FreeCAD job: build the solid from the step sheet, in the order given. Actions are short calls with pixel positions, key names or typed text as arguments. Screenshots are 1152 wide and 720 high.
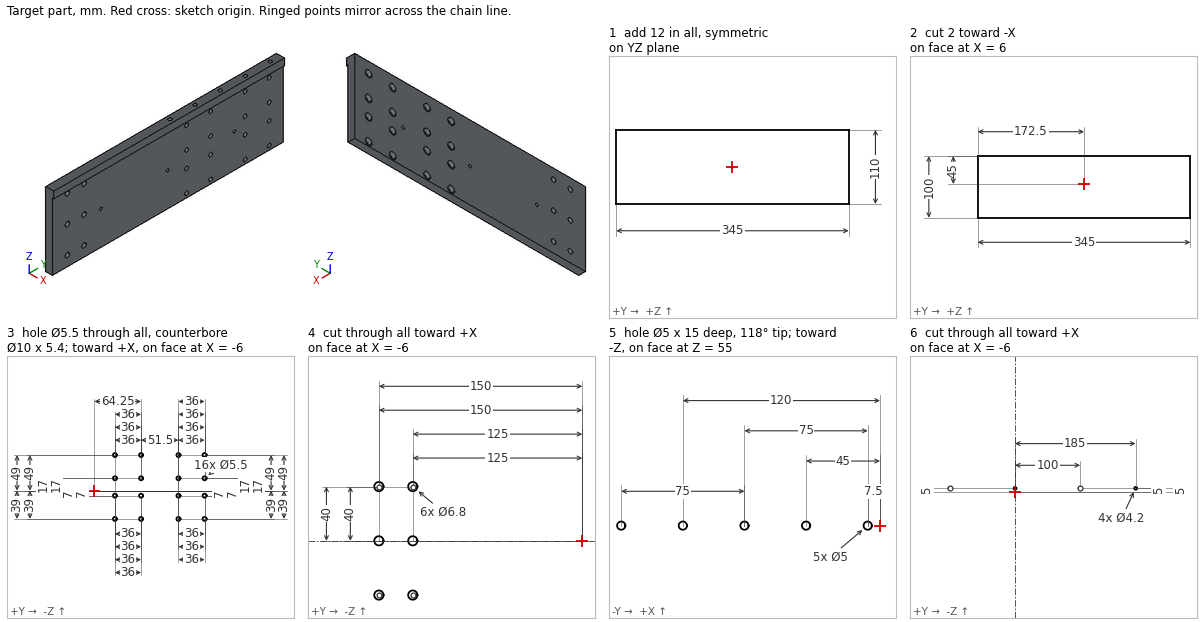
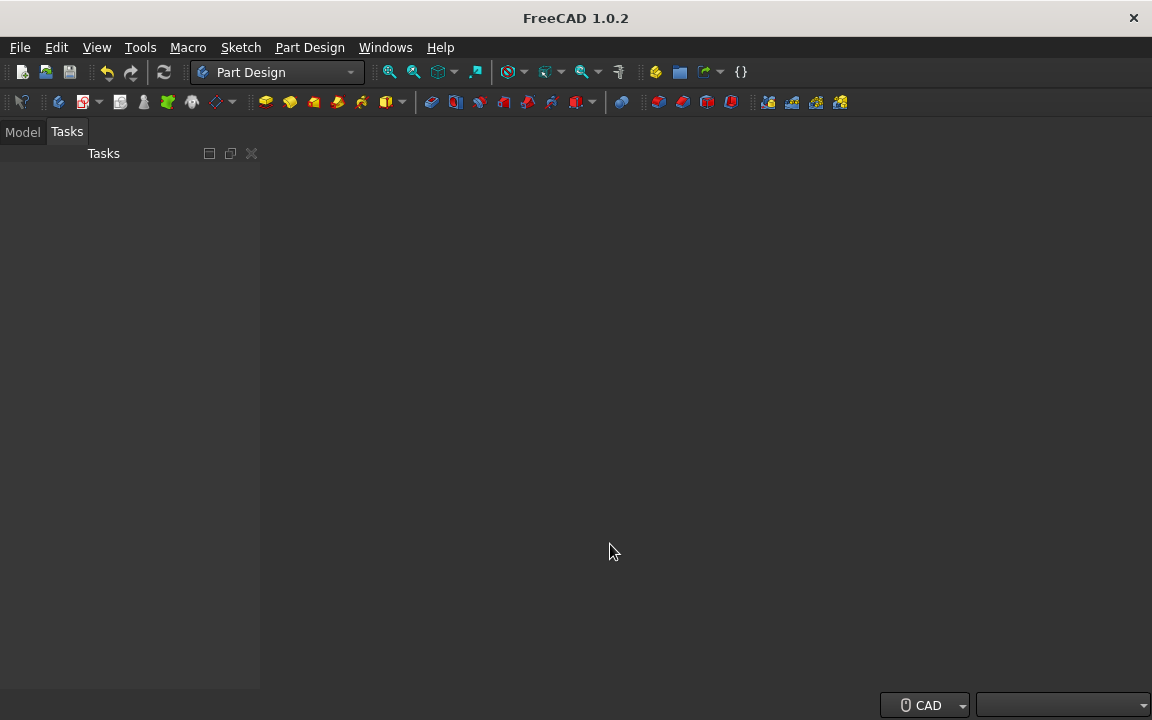
click(22, 72)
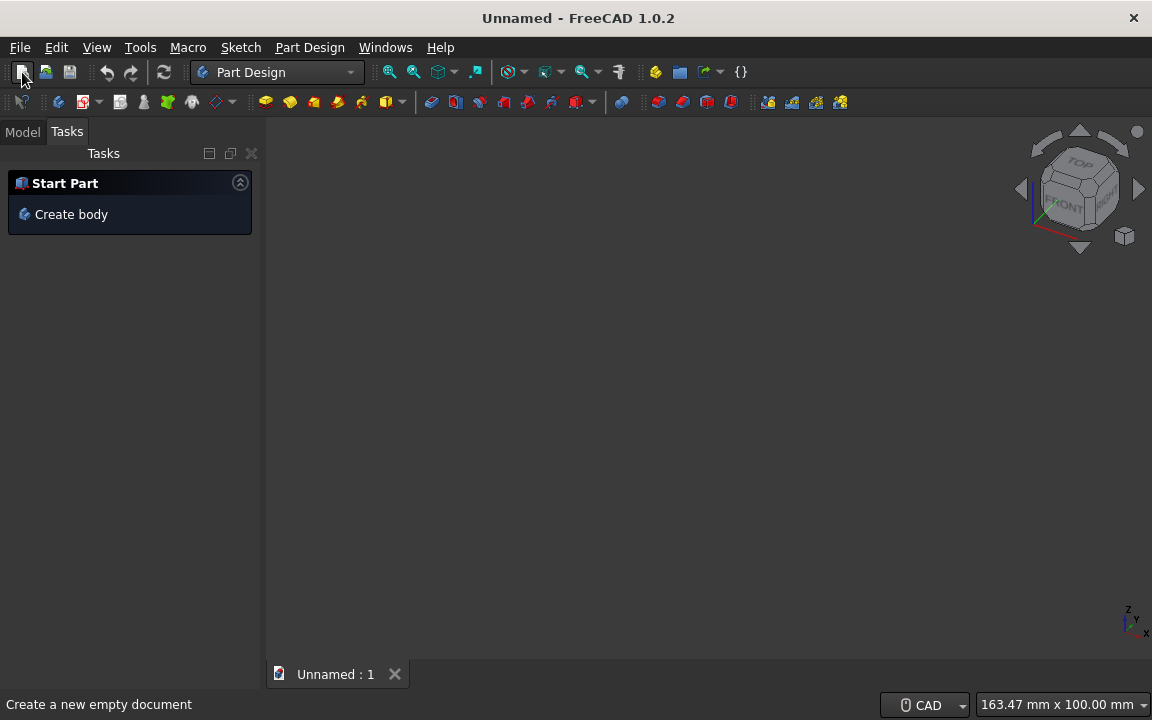
click(84, 102)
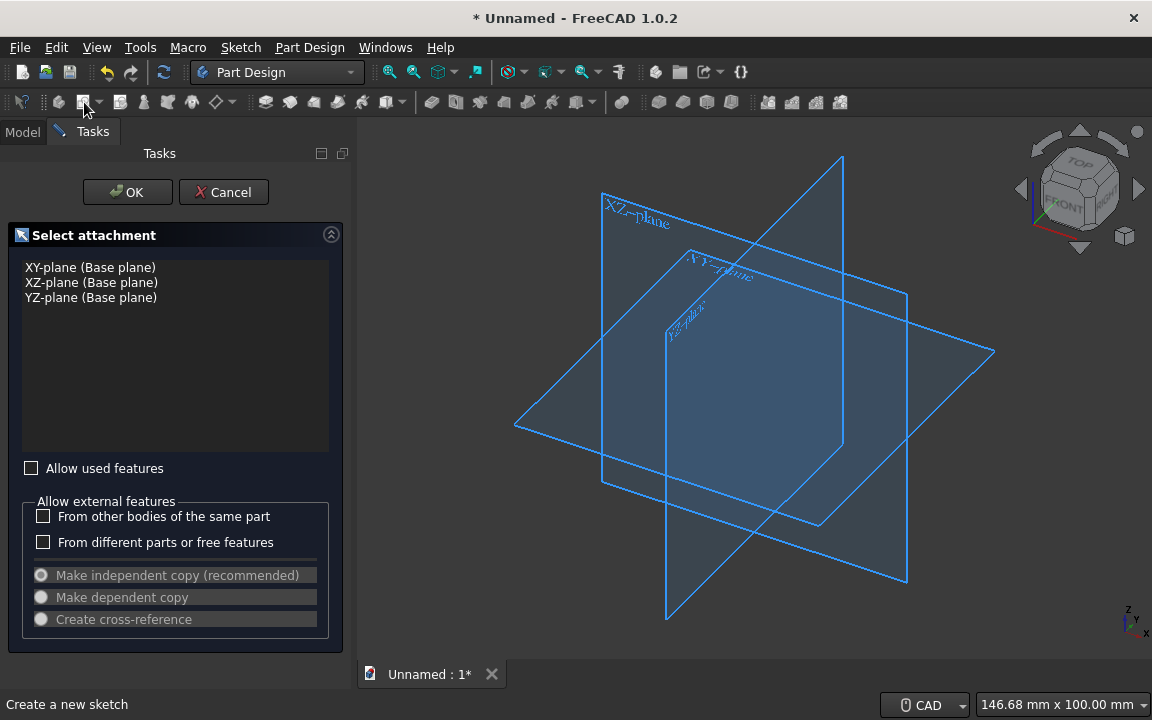
click(82, 298)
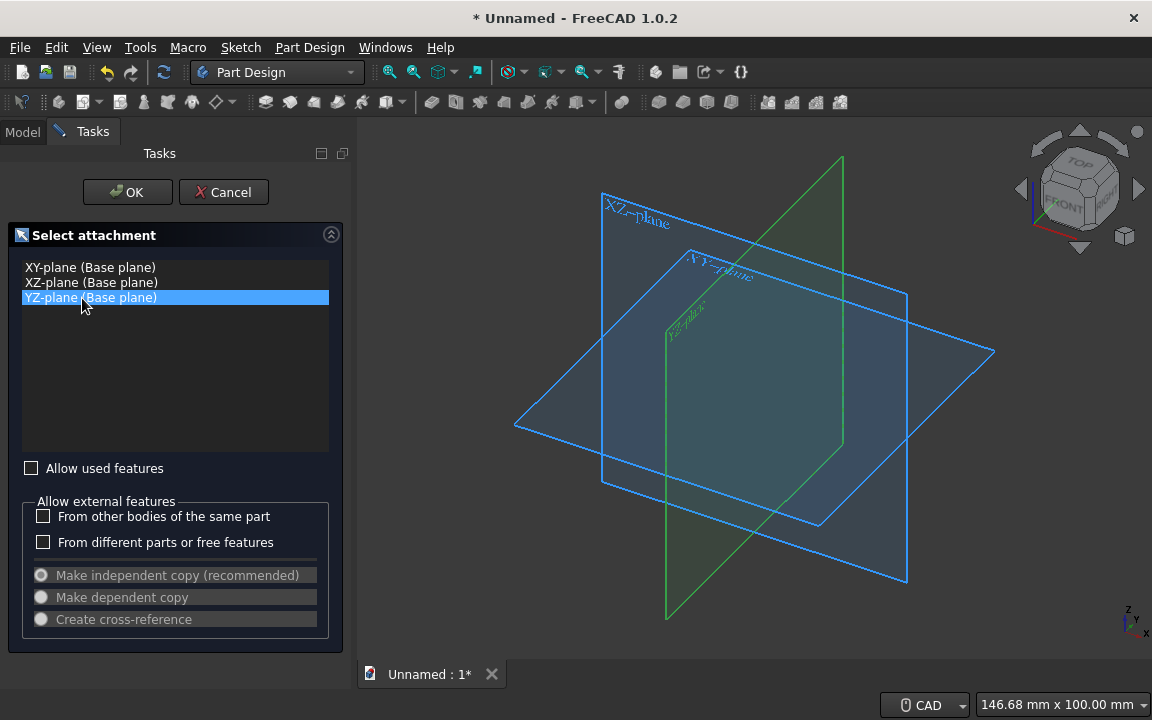
click(128, 192)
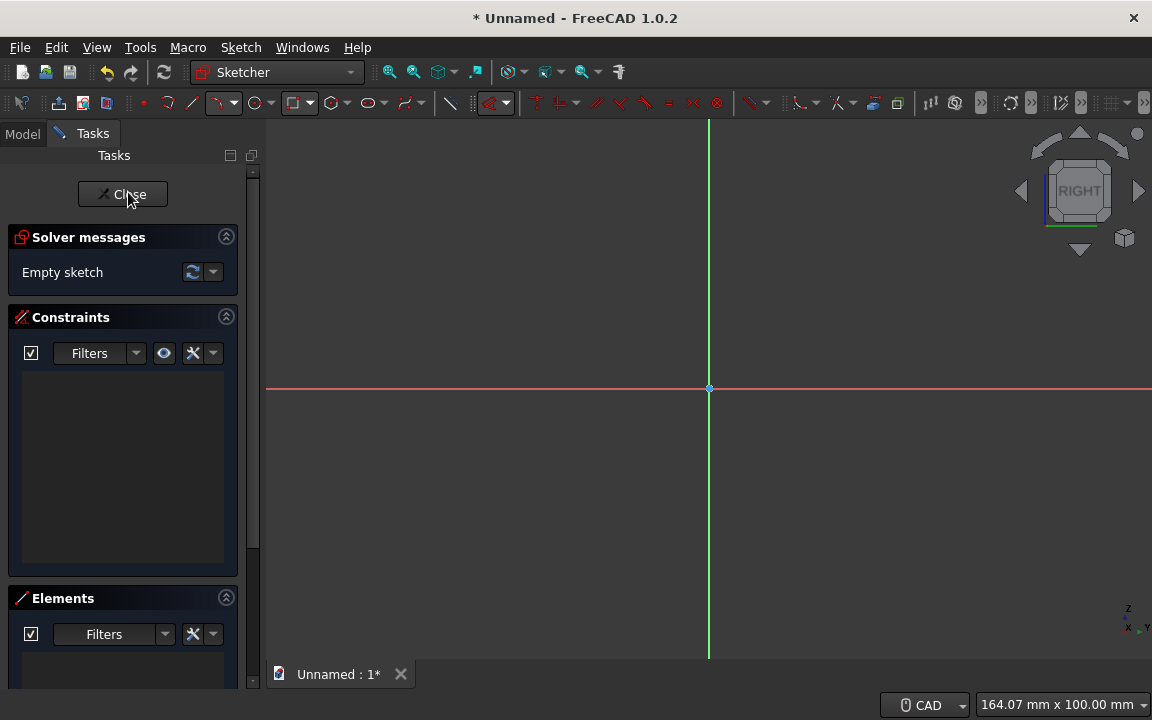
scroll(618, 389, down, 7)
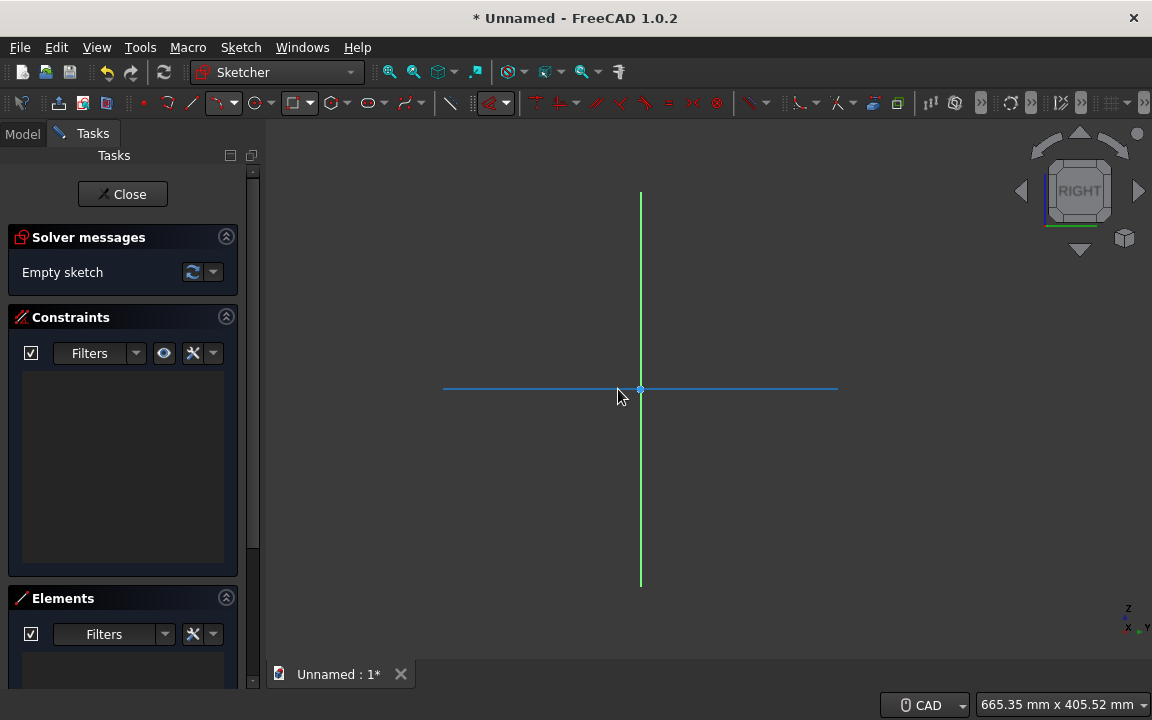
key(g)
key(v)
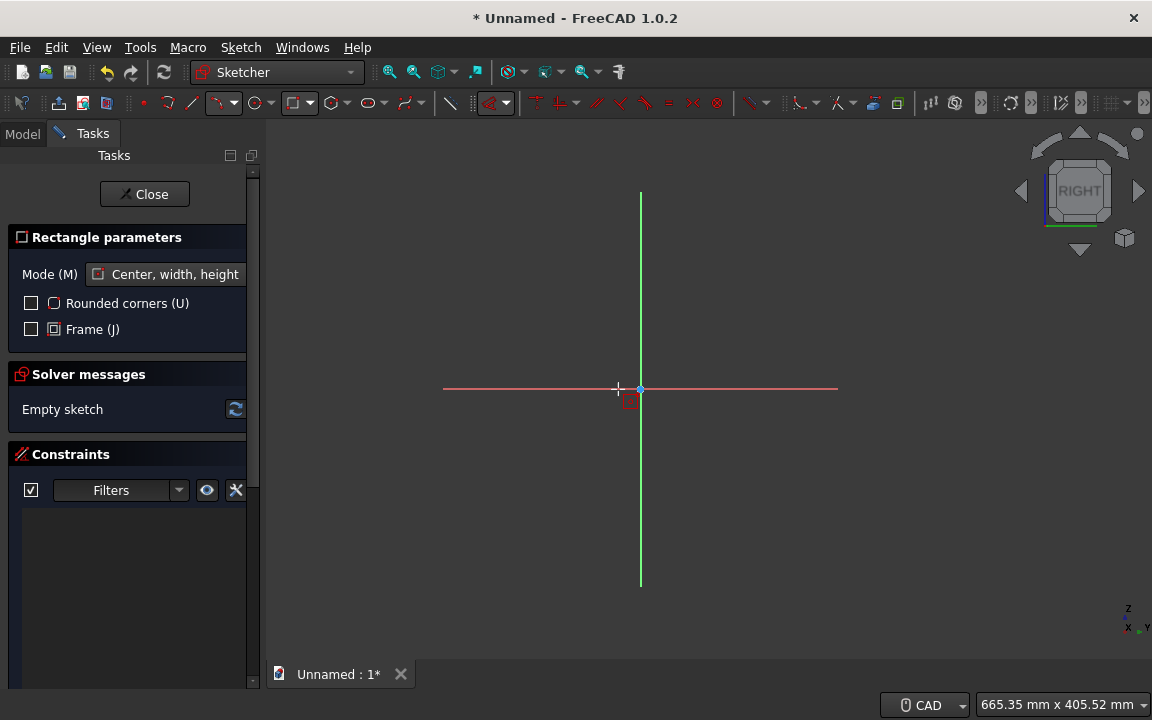
click(641, 389)
click(870, 316)
key(Escape)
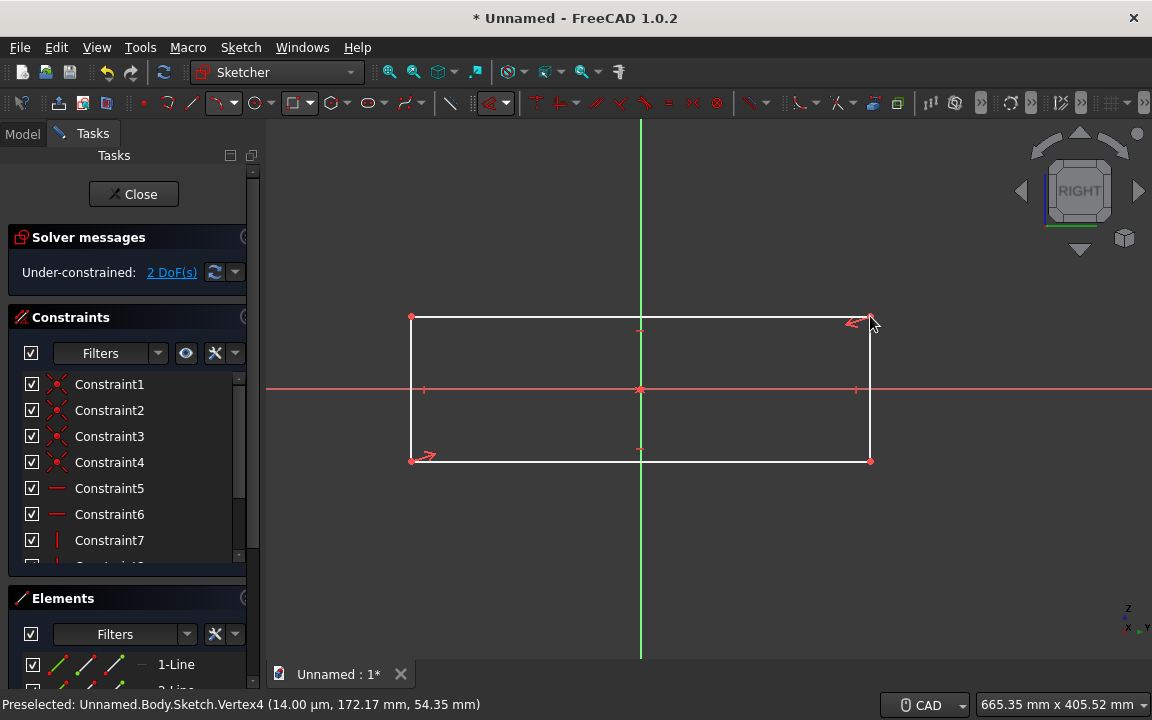
click(549, 462)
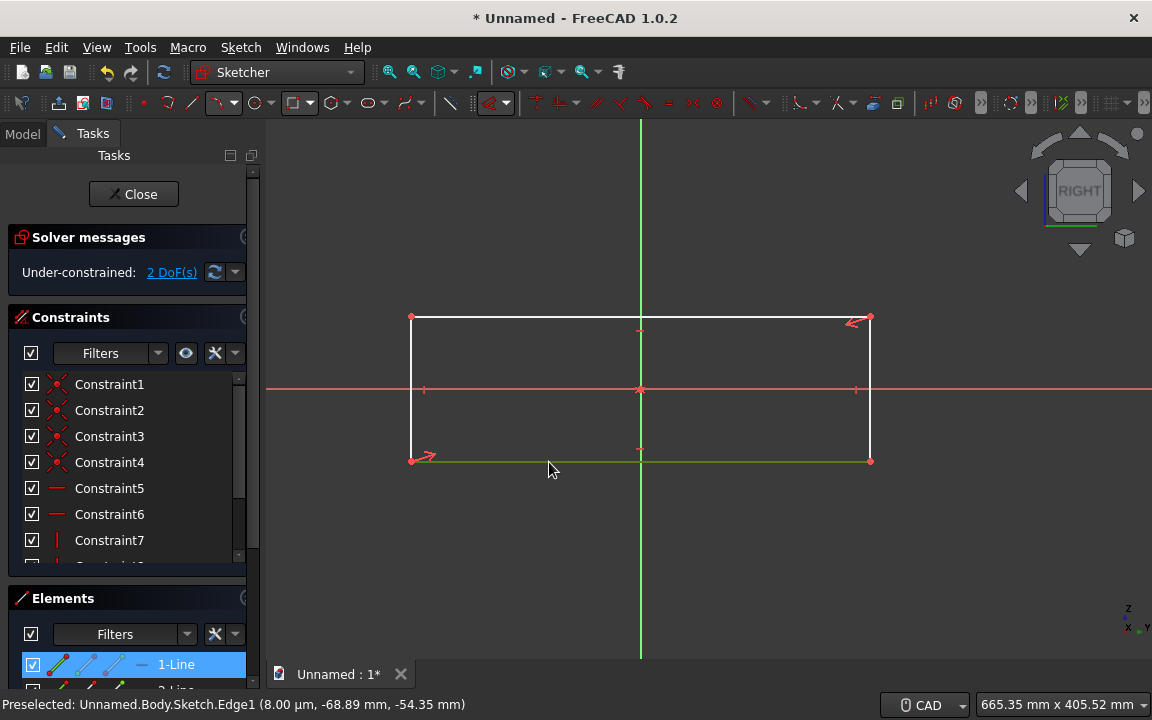
key(l)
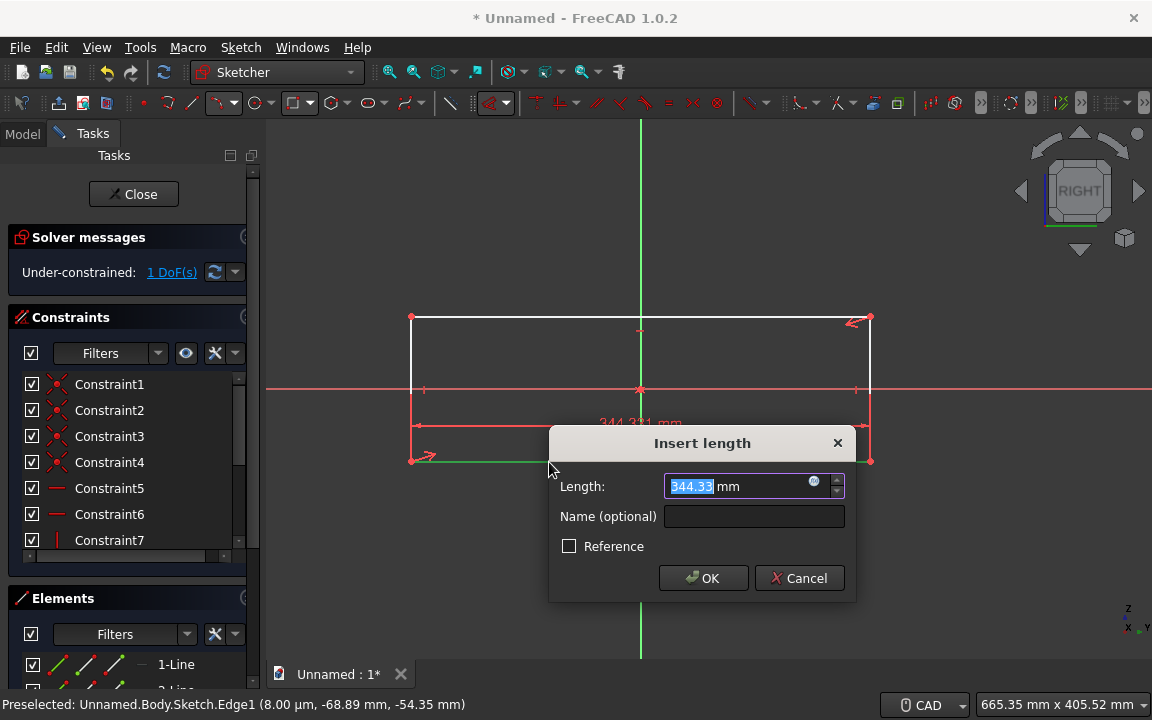
text(345)
key(Return)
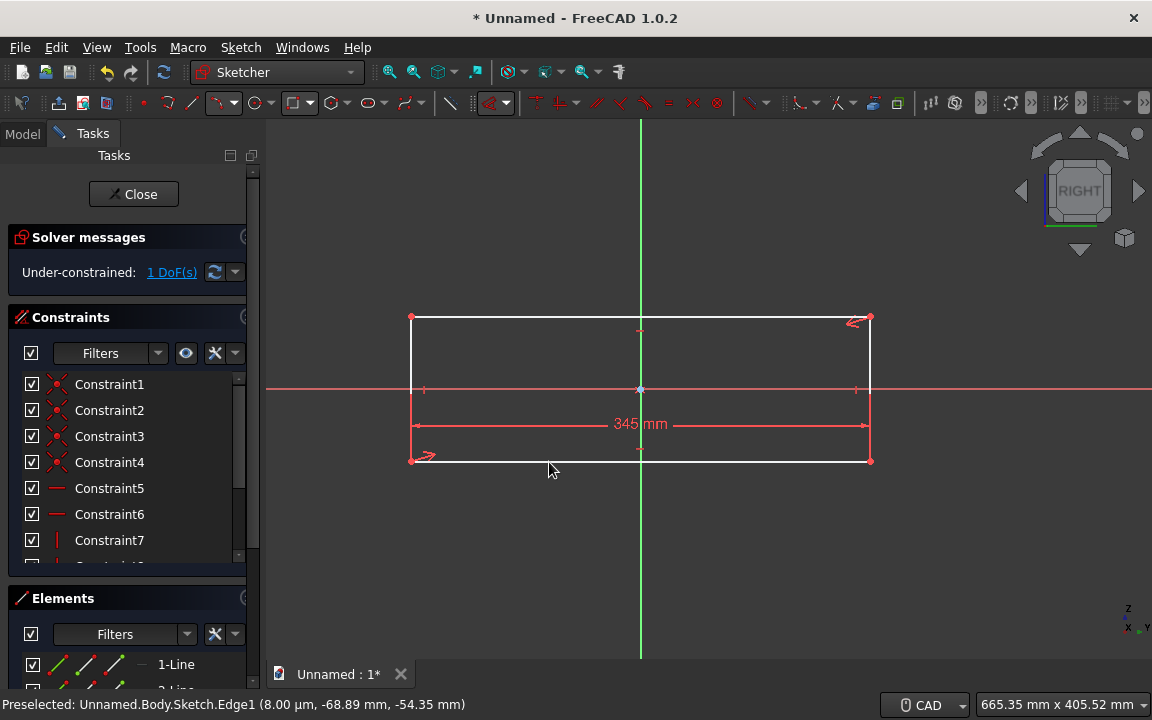
click(870, 418)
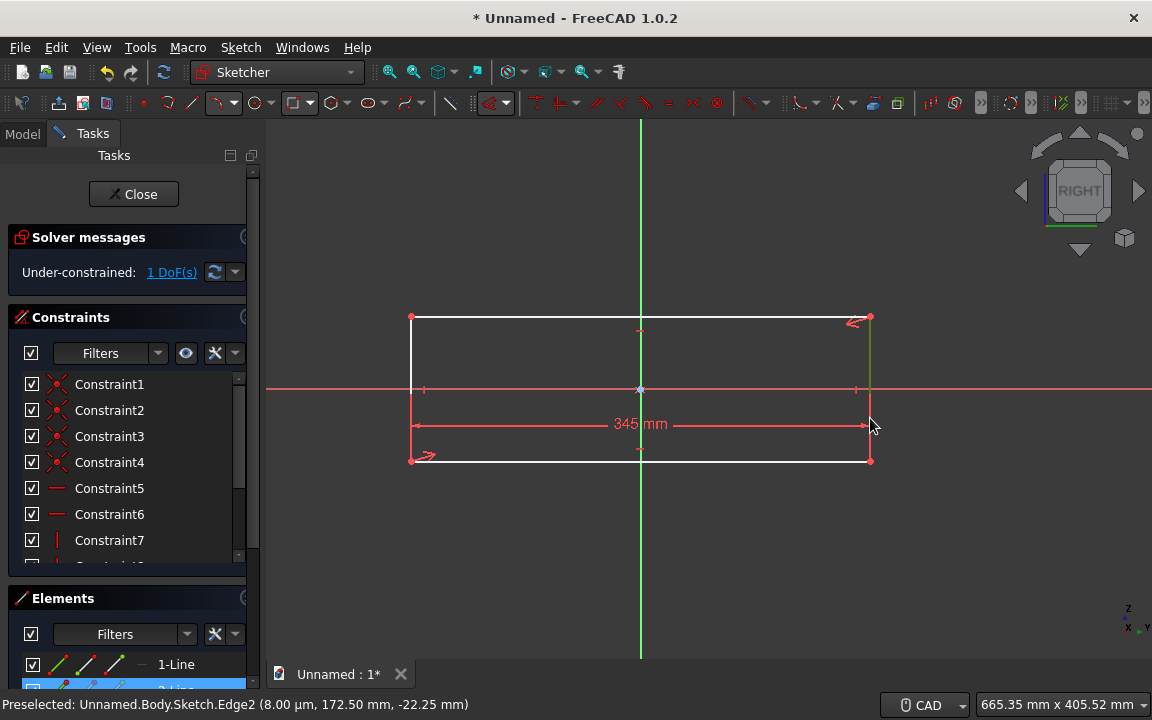
key(i)